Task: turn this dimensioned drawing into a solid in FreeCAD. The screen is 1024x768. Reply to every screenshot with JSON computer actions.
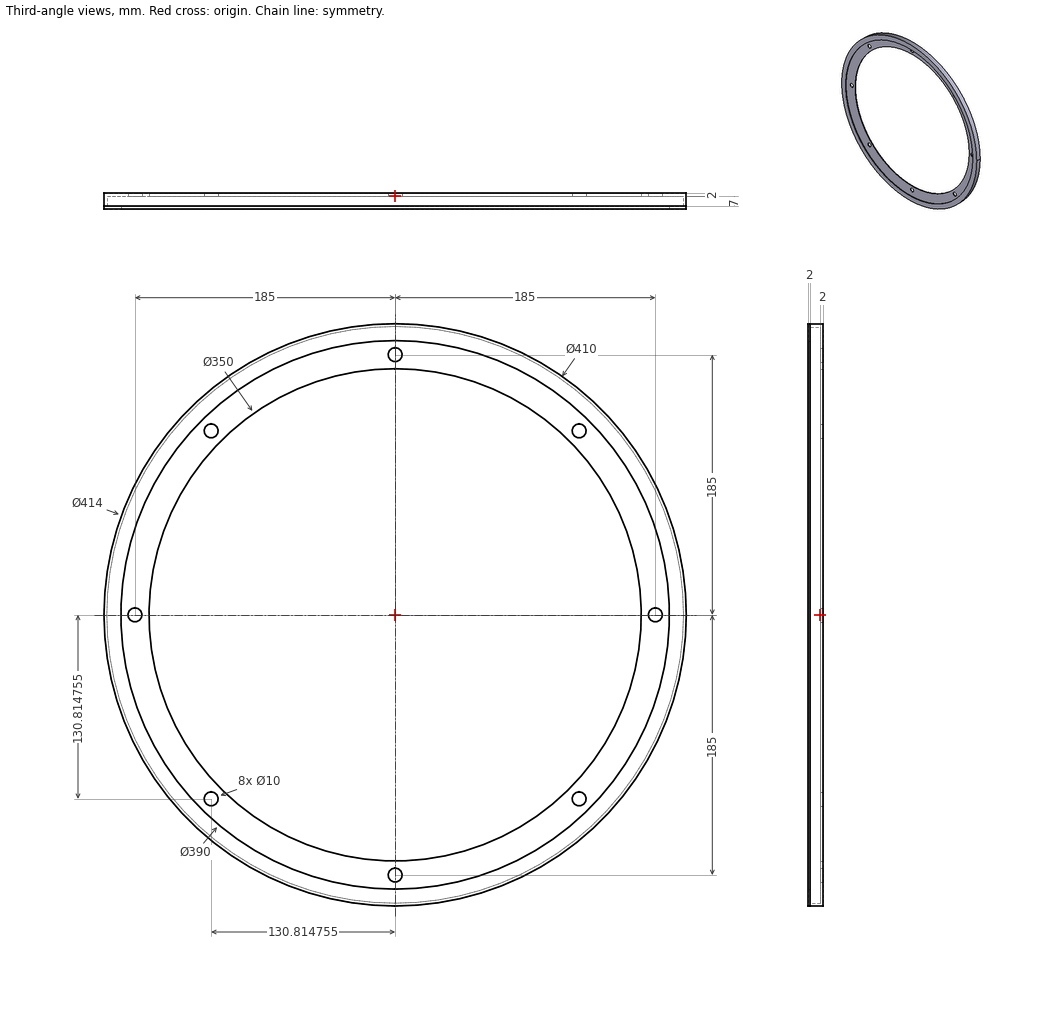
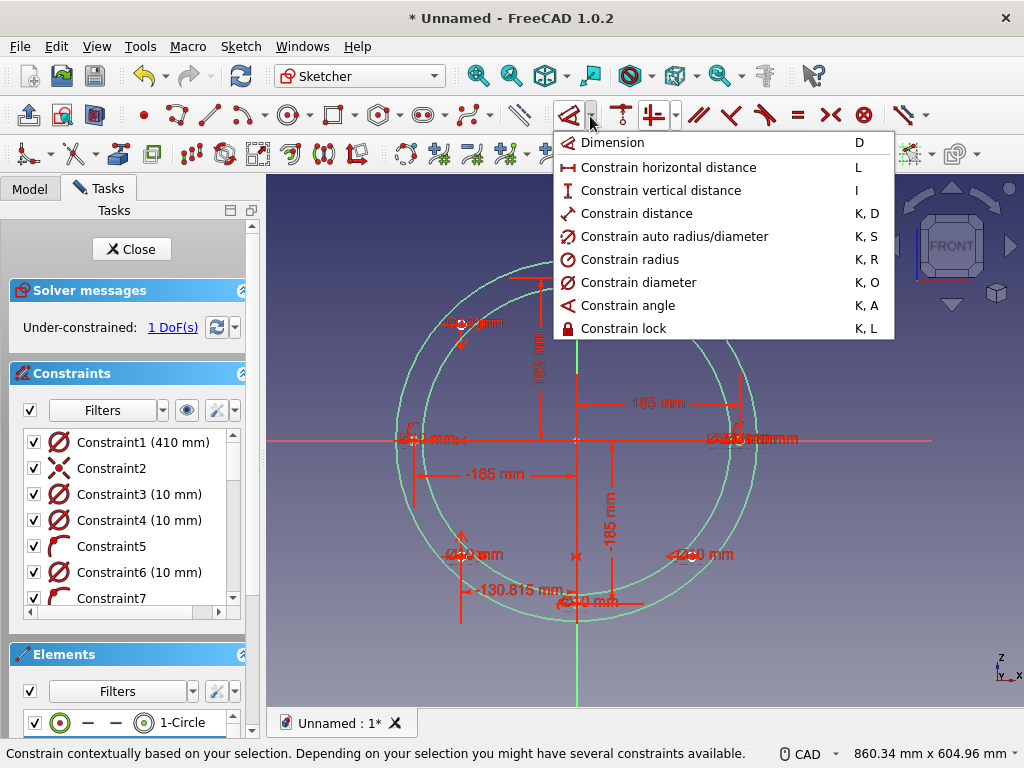
{"action": "left_click", "coordinate": [724, 190]}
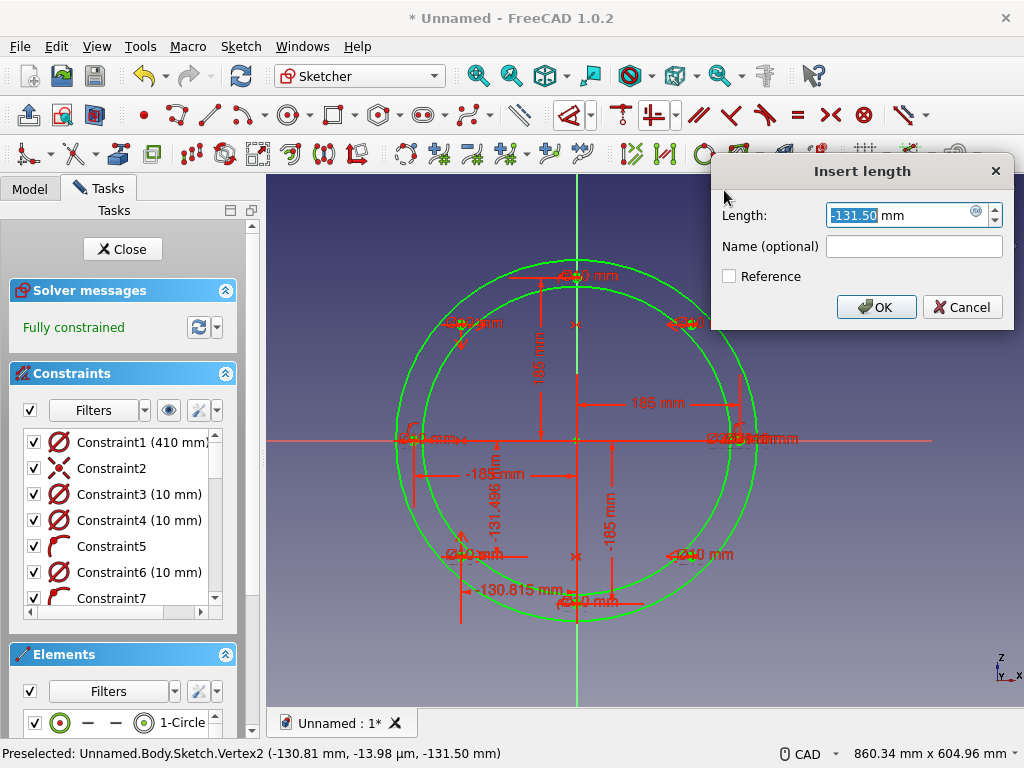
{"action": "type", "text": "-130.814755"}
{"action": "key", "text": "Return"}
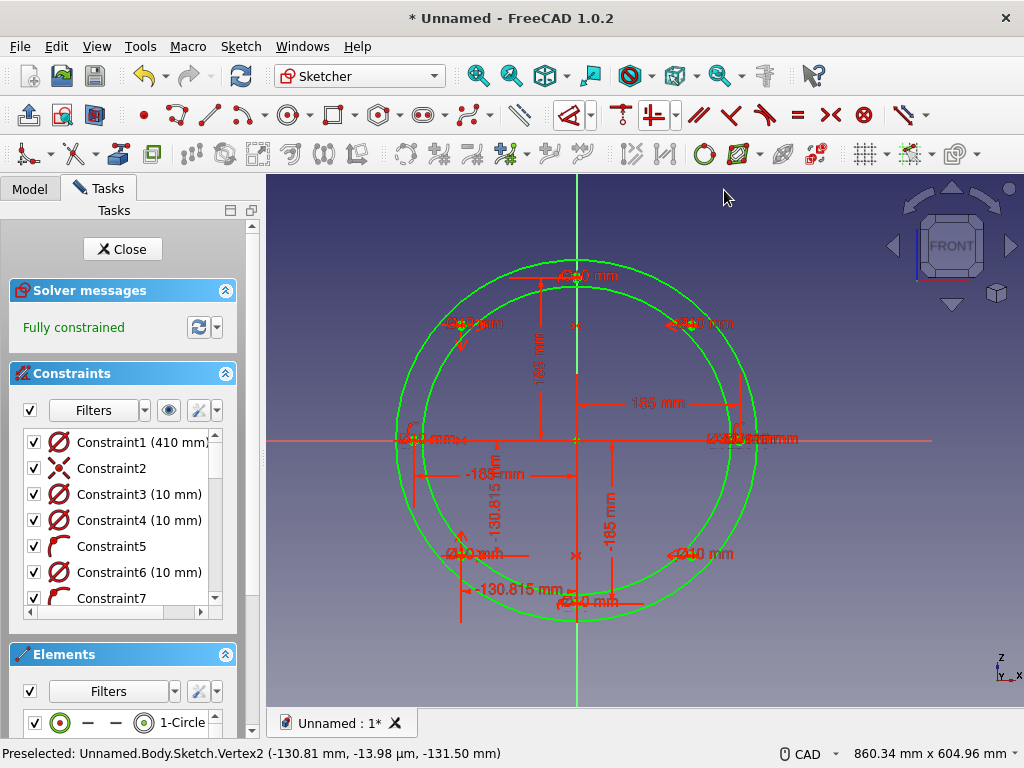
{"action": "left_click", "coordinate": [123, 249]}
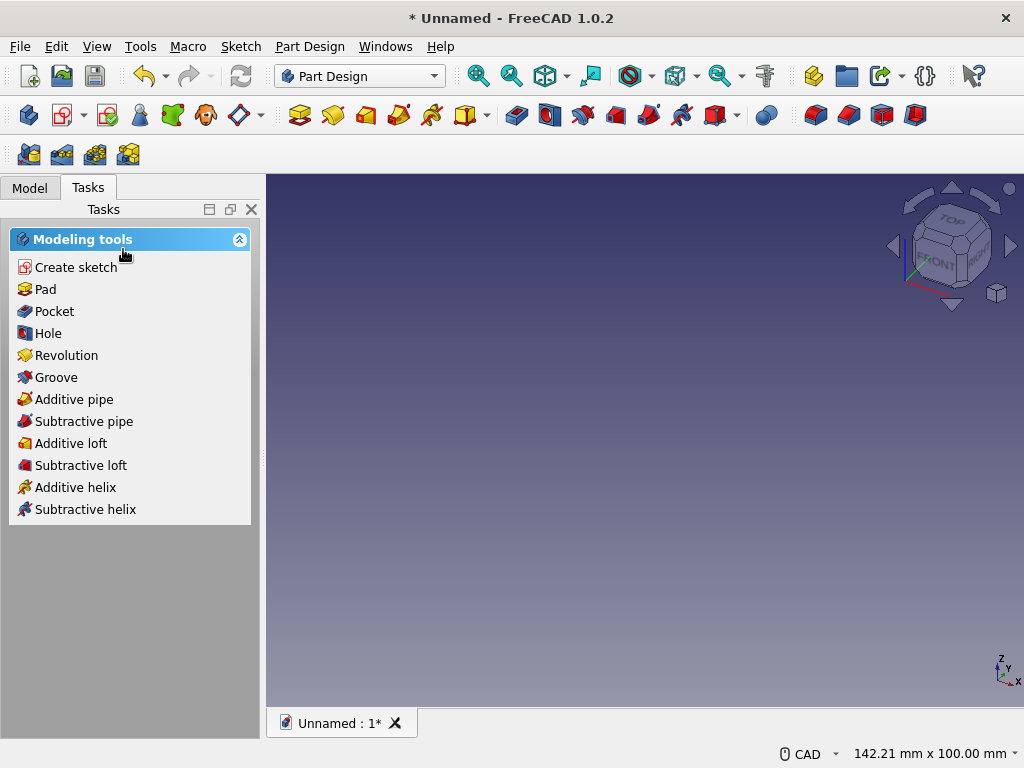
{"action": "left_click", "coordinate": [300, 116]}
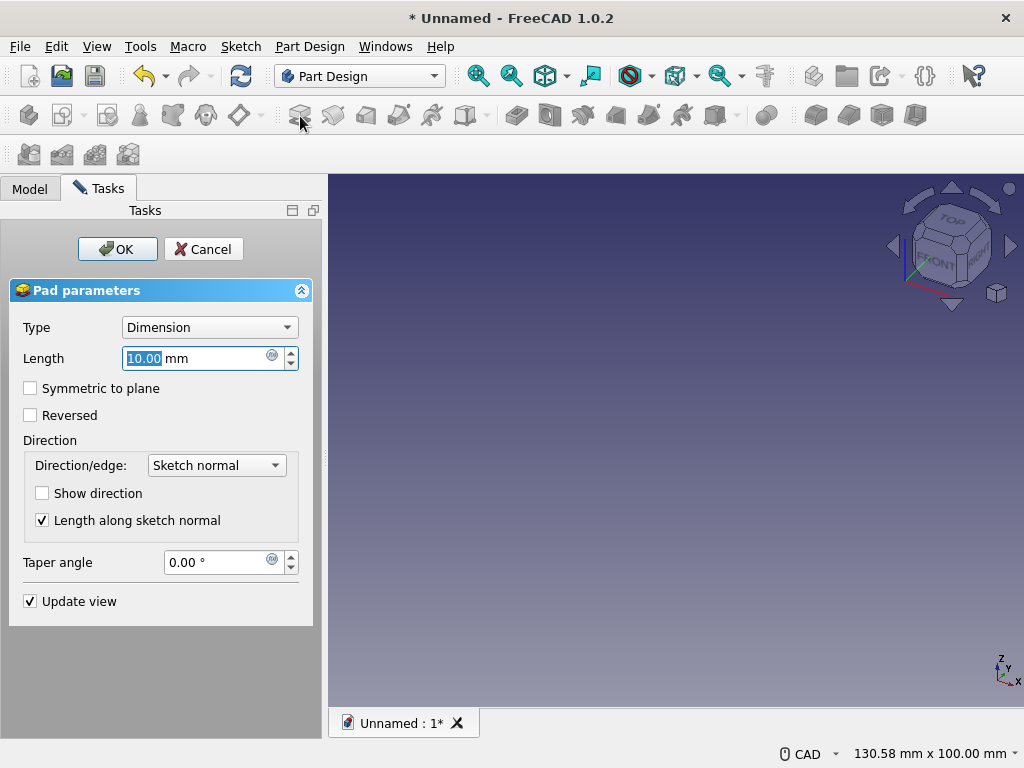
{"action": "type", "text": "2"}
{"action": "key", "text": "Tab"}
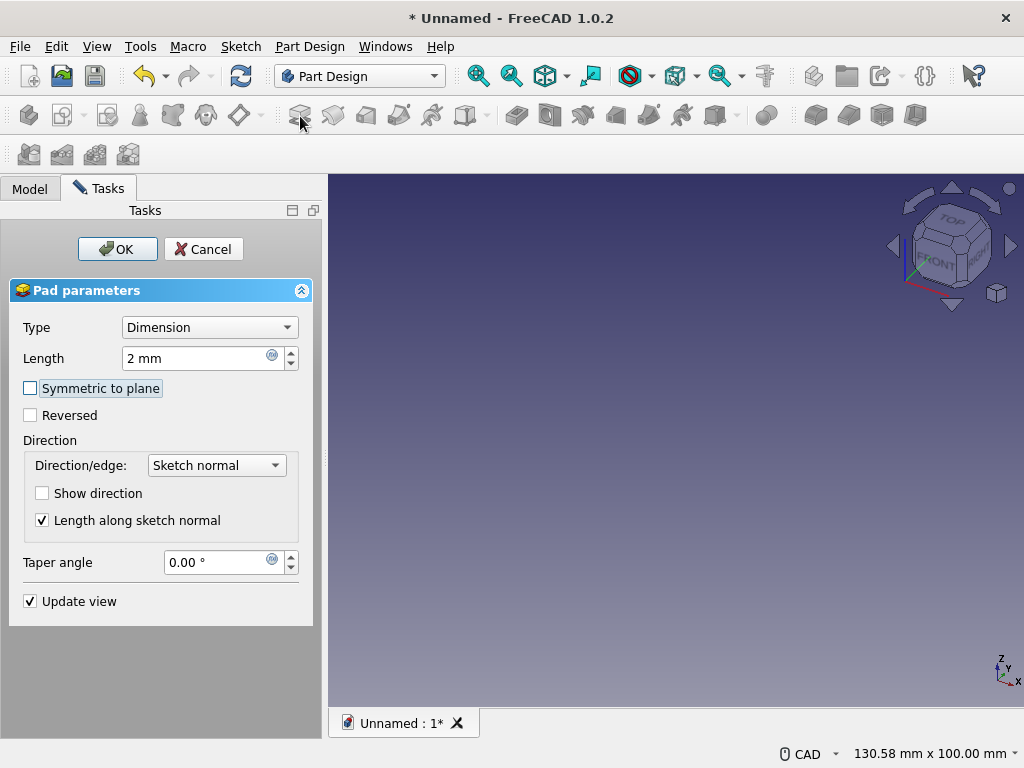
{"action": "left_click", "coordinate": [31, 415]}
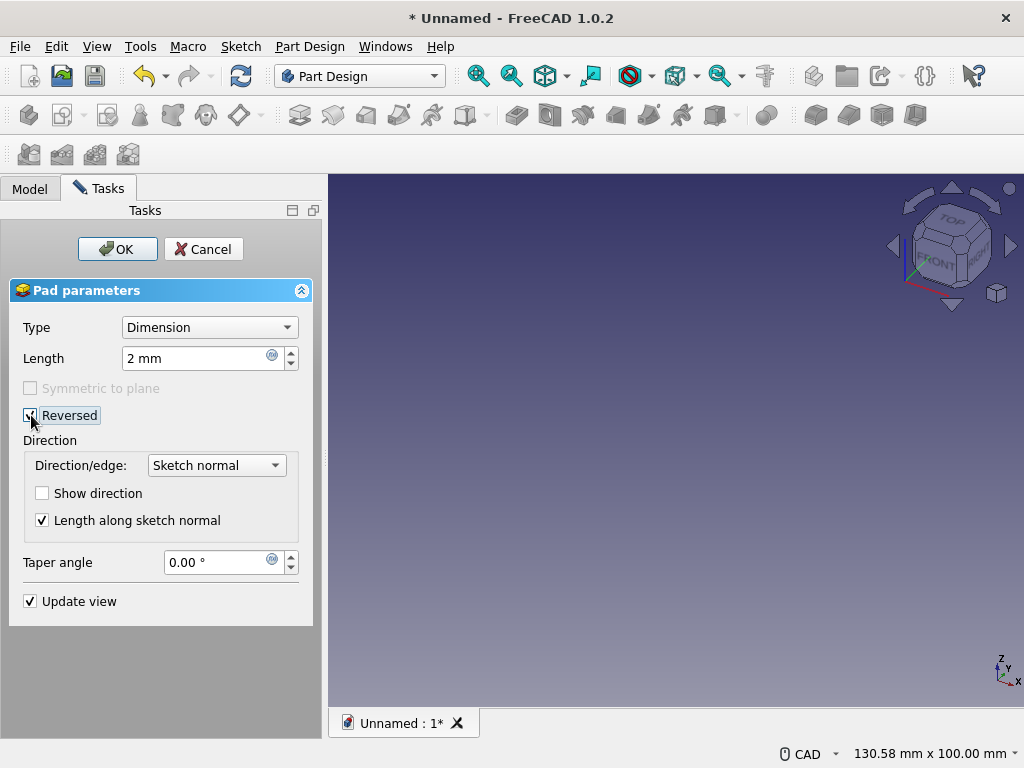
{"action": "left_click", "coordinate": [118, 249]}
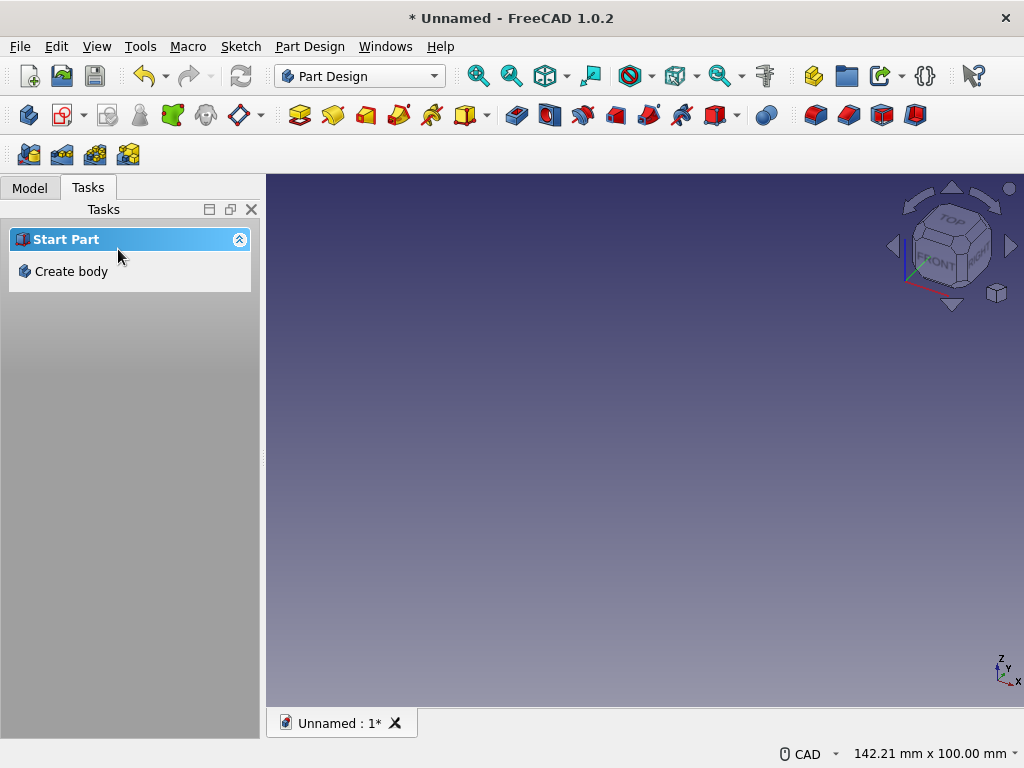
{"action": "left_click", "coordinate": [479, 76]}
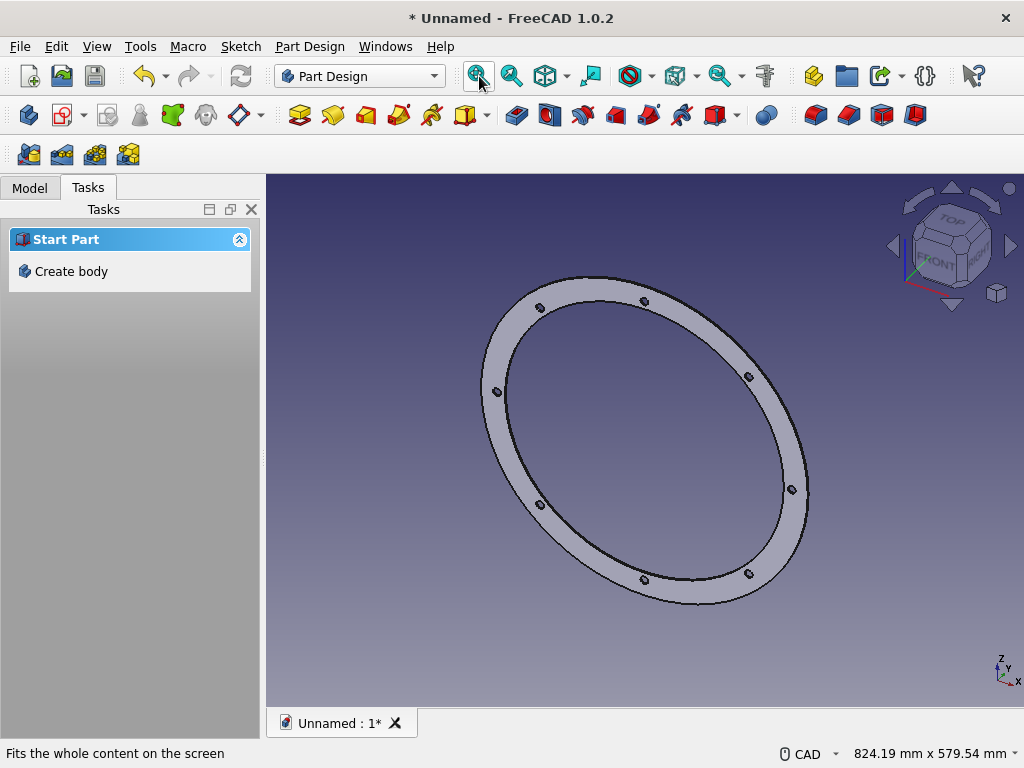
{"action": "left_click", "coordinate": [62, 116]}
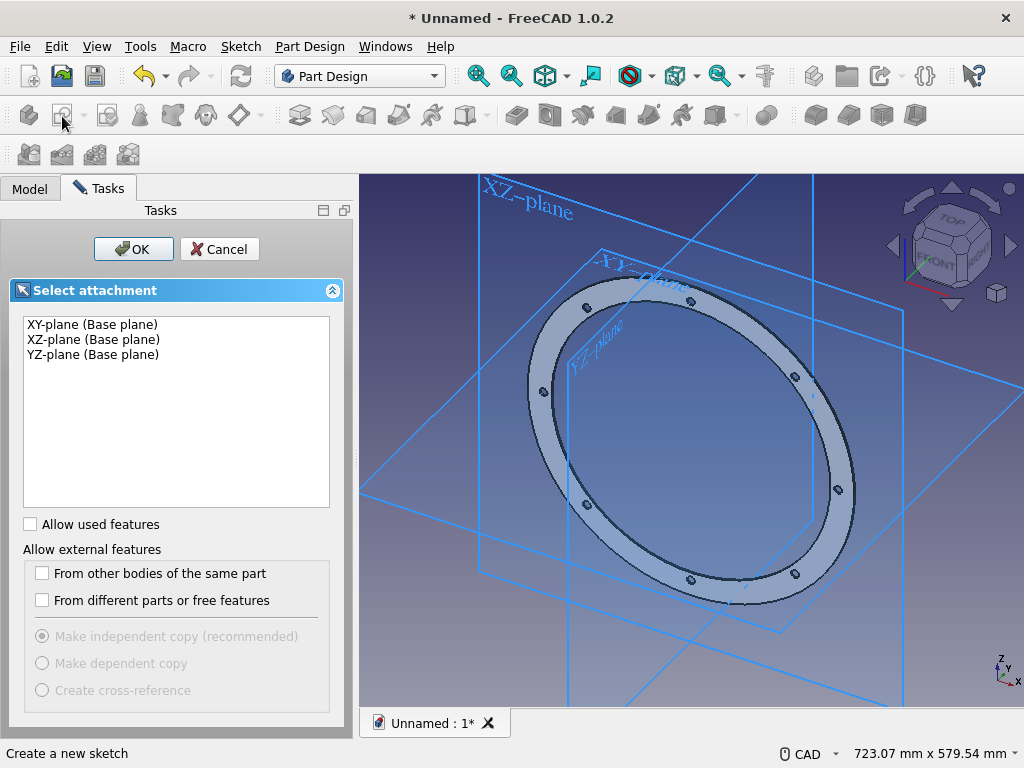
{"action": "left_click", "coordinate": [84, 340]}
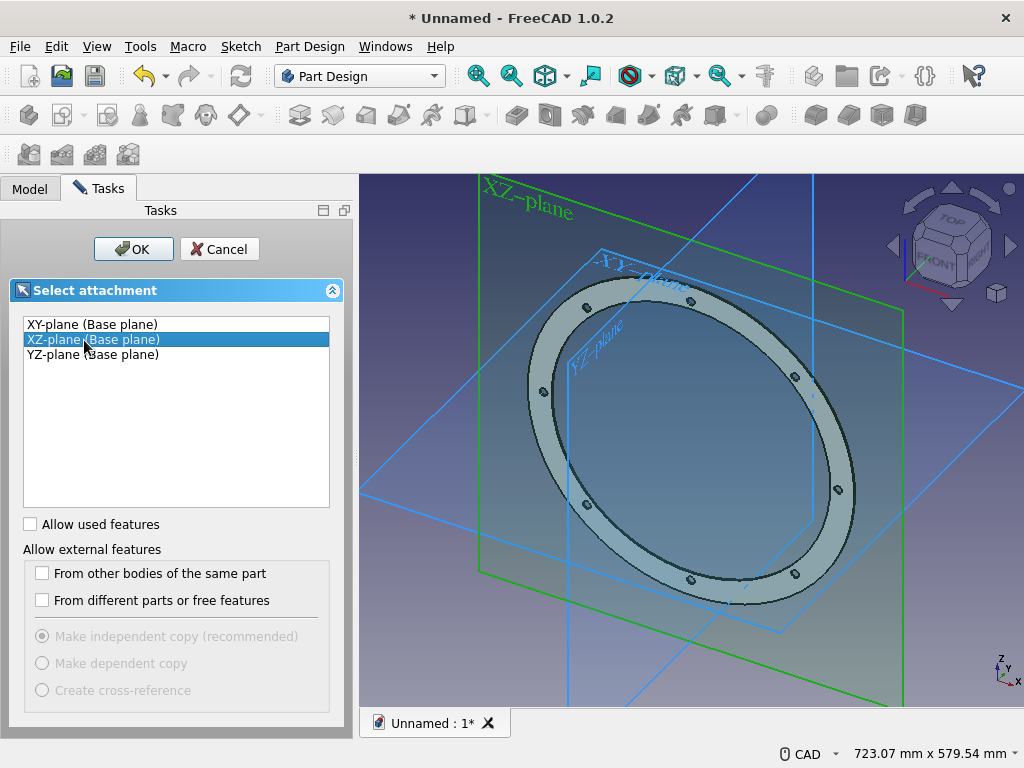
{"action": "left_click", "coordinate": [134, 249]}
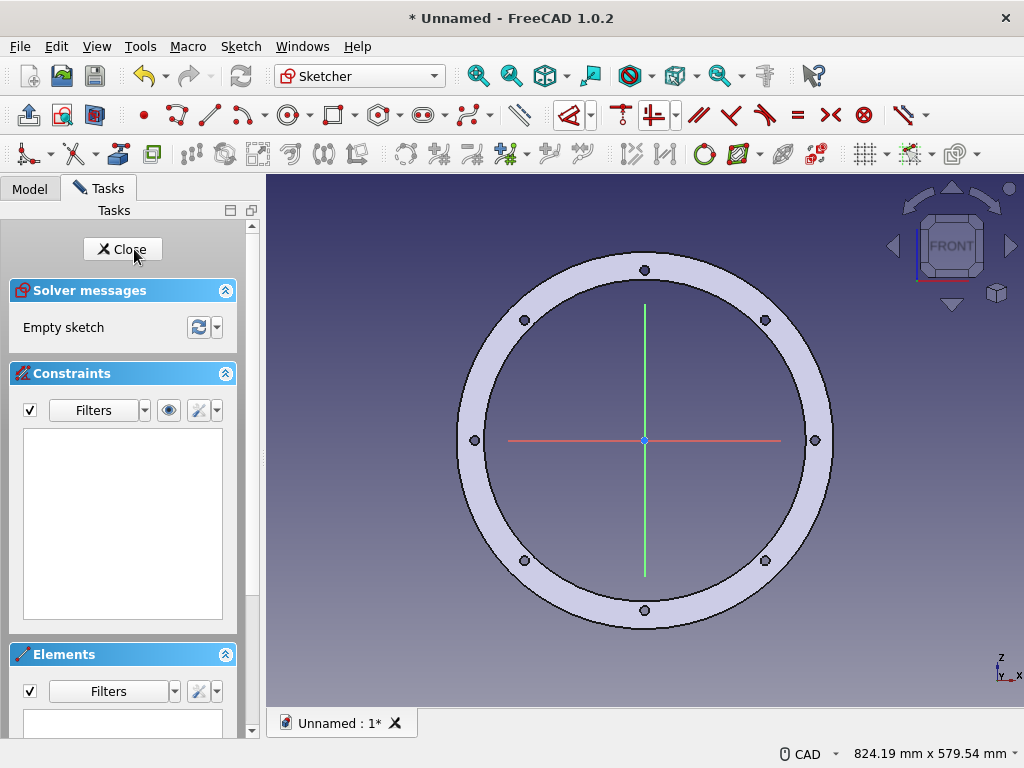
{"action": "scroll", "coordinate": [294, 440], "scroll_direction": "down", "scroll_amount": 1}